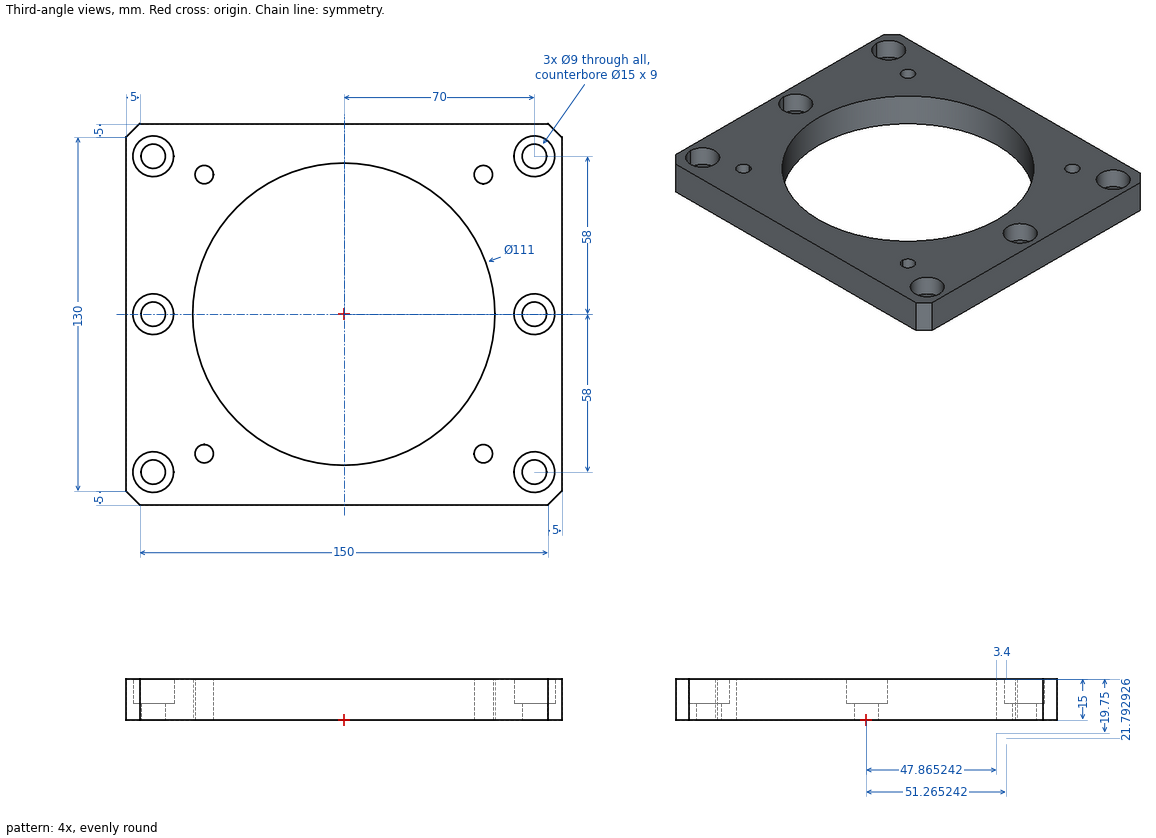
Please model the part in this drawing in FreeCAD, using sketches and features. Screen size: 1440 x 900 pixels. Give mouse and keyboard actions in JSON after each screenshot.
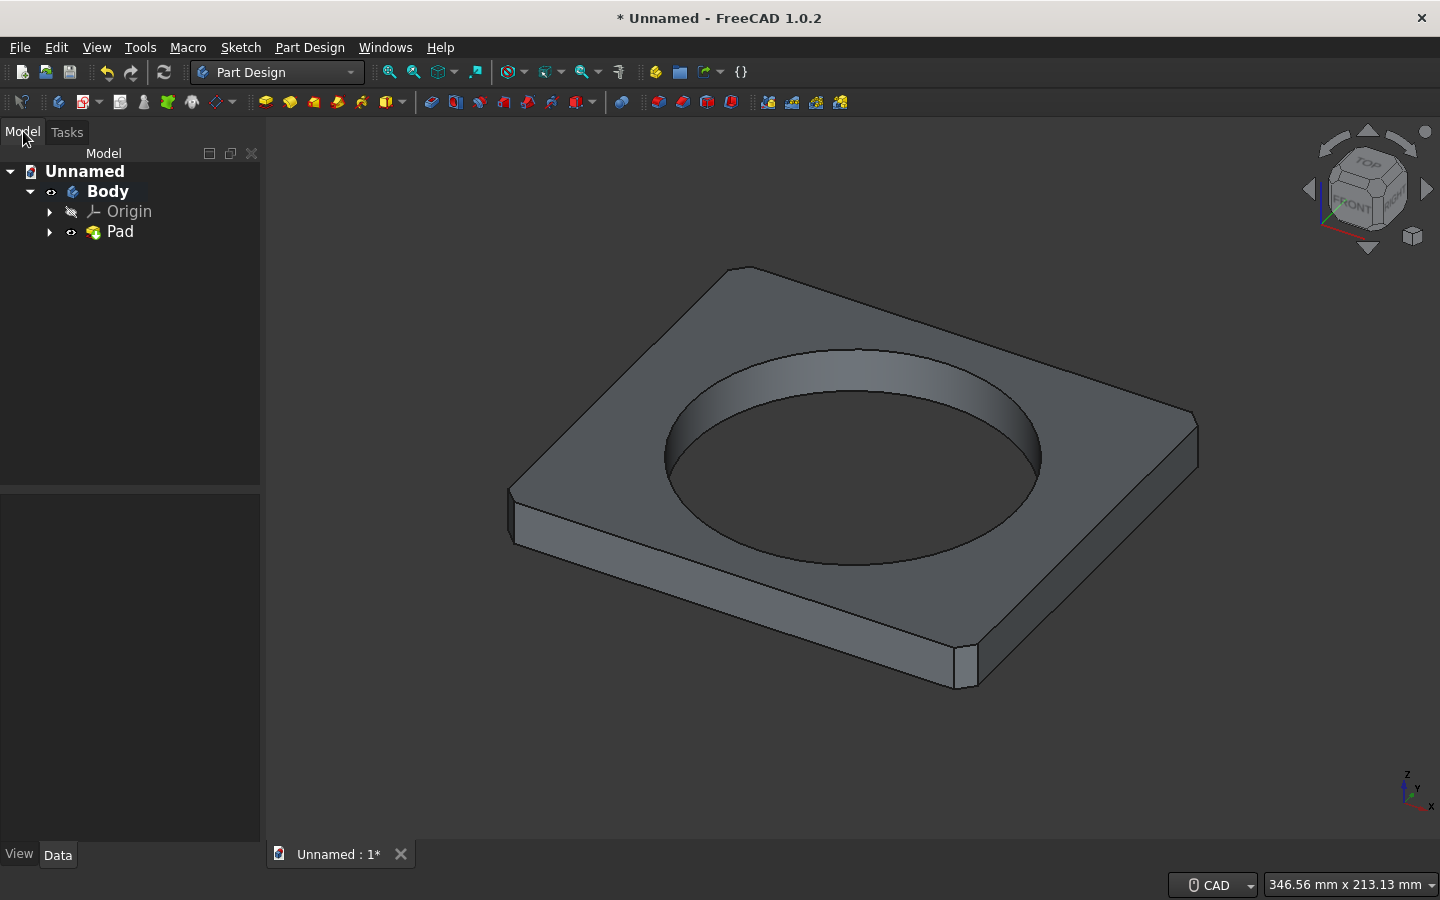
{"action": "left_click", "coordinate": [50, 212]}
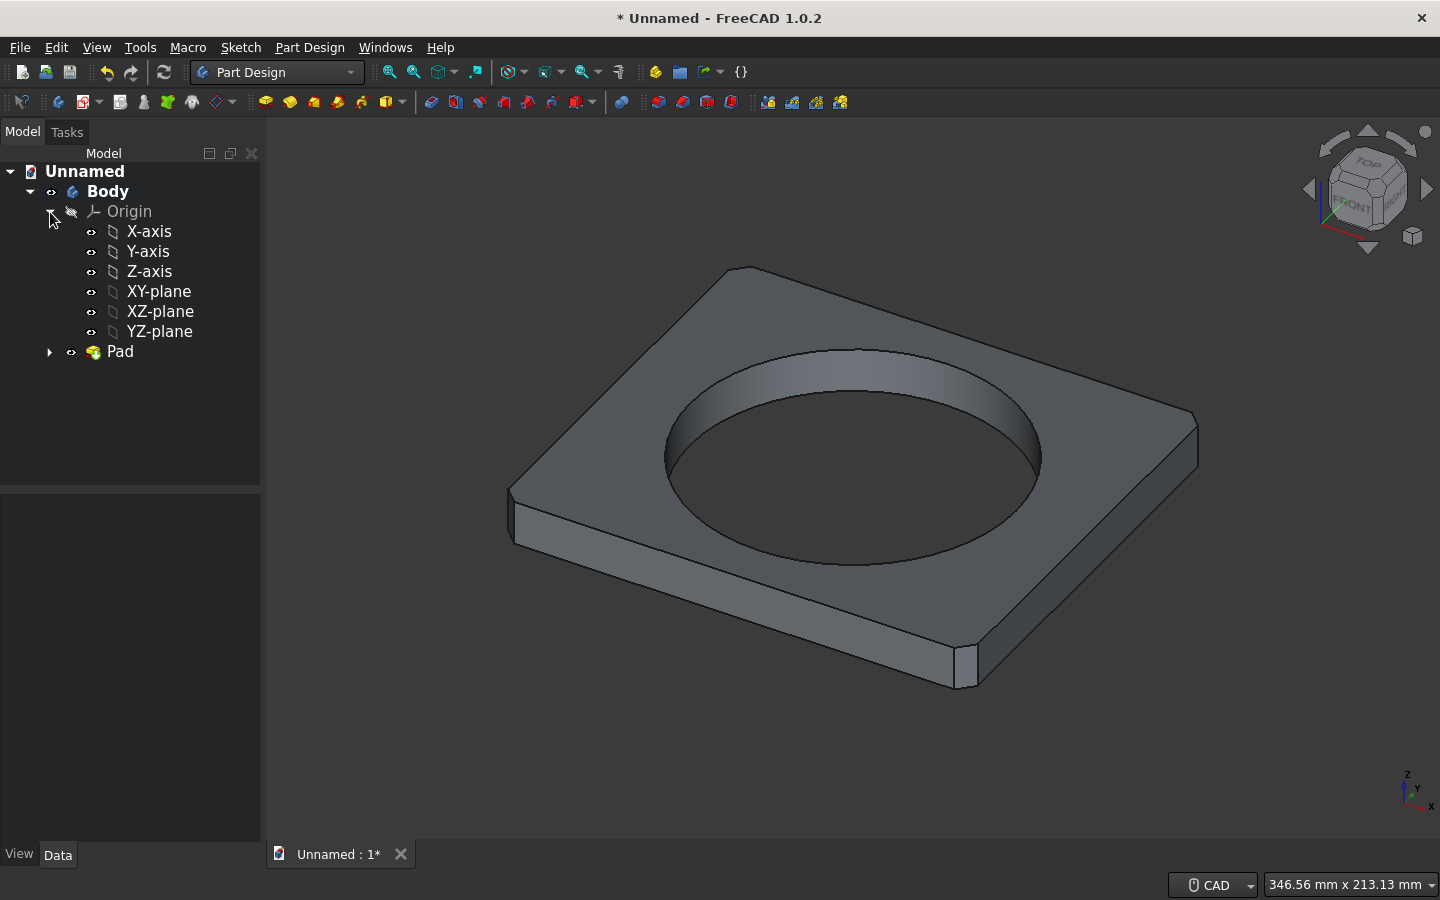
{"action": "left_click", "coordinate": [136, 332]}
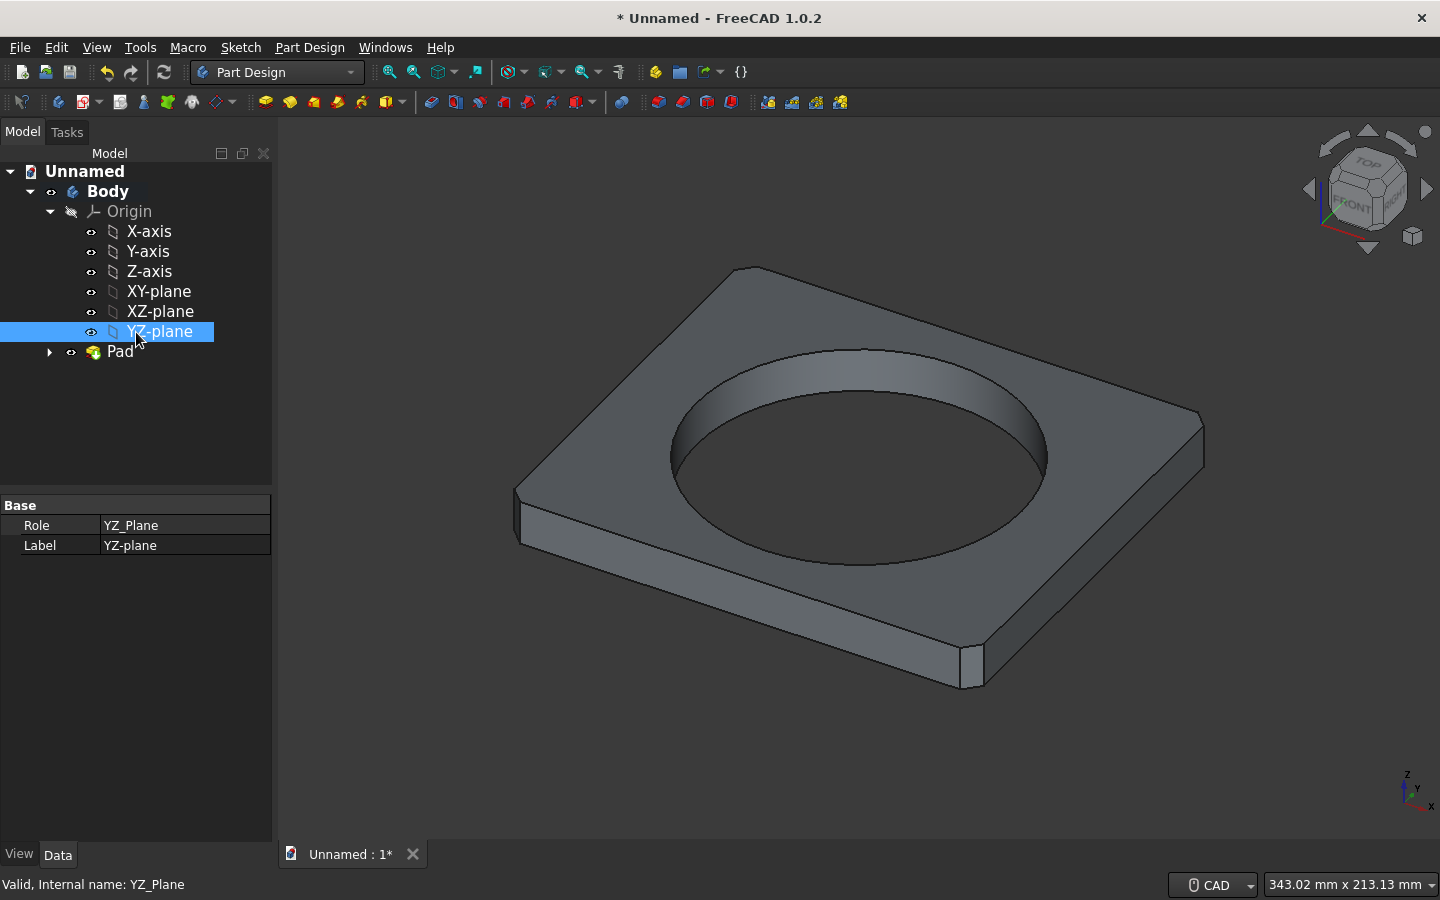
{"action": "left_click", "coordinate": [216, 102]}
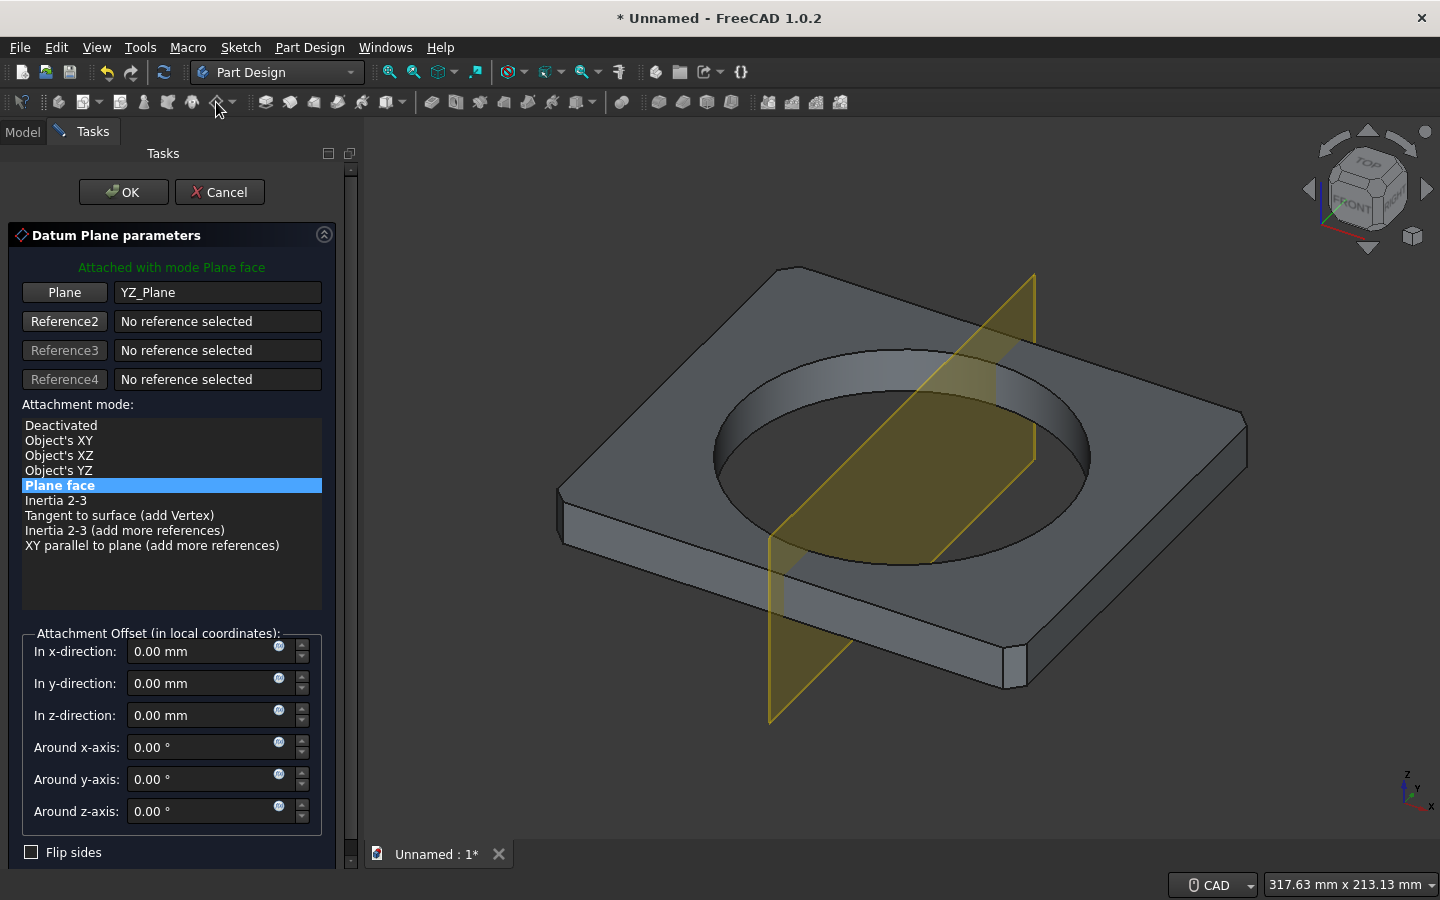
{"action": "triple_click", "coordinate": [210, 715]}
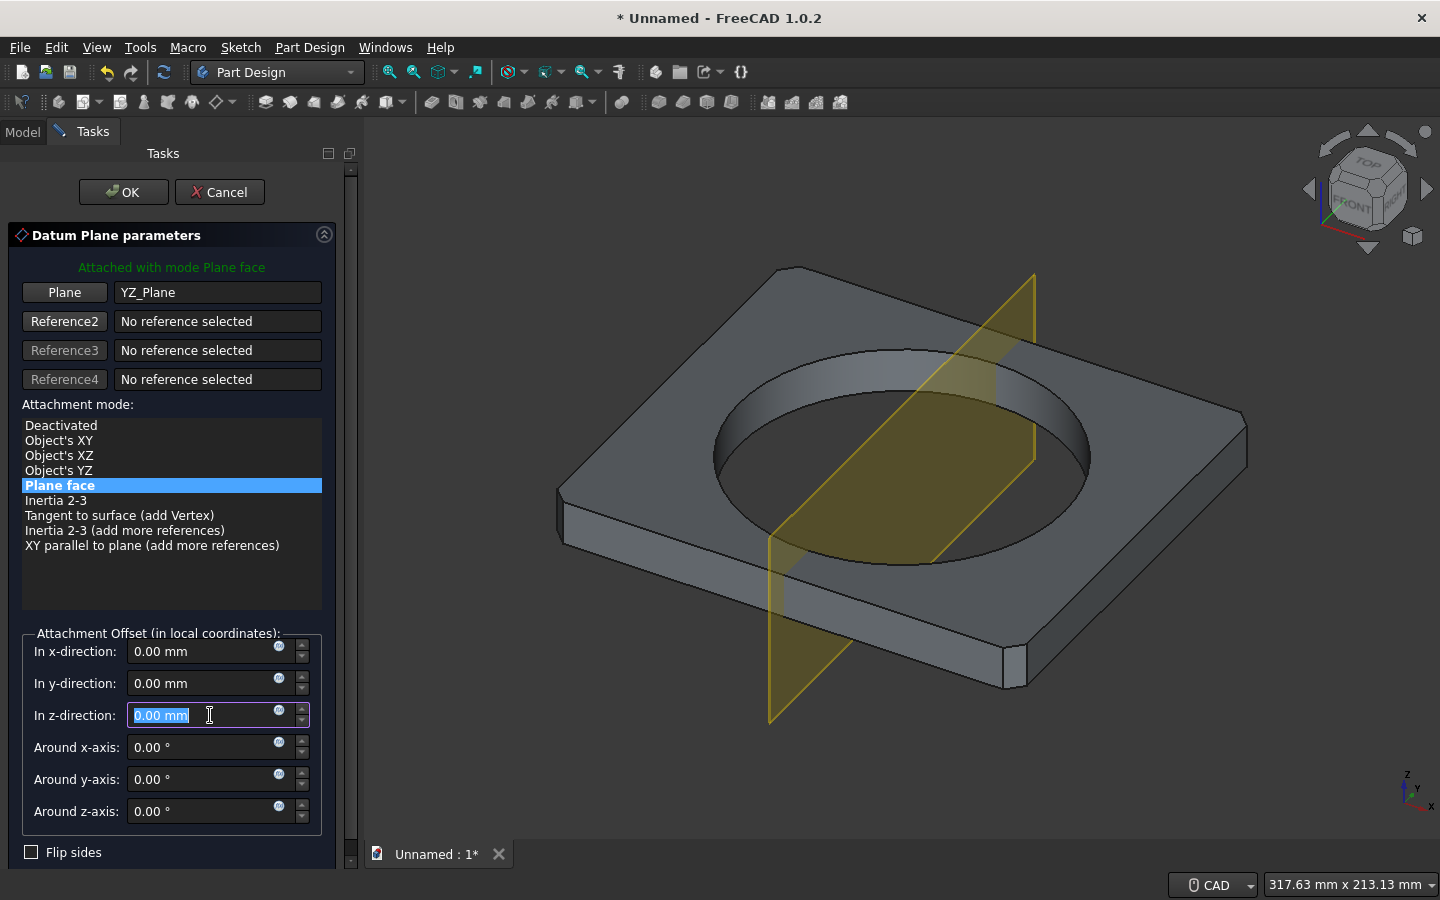
{"action": "type", "text": "51.265242"}
{"action": "key", "text": "Tab"}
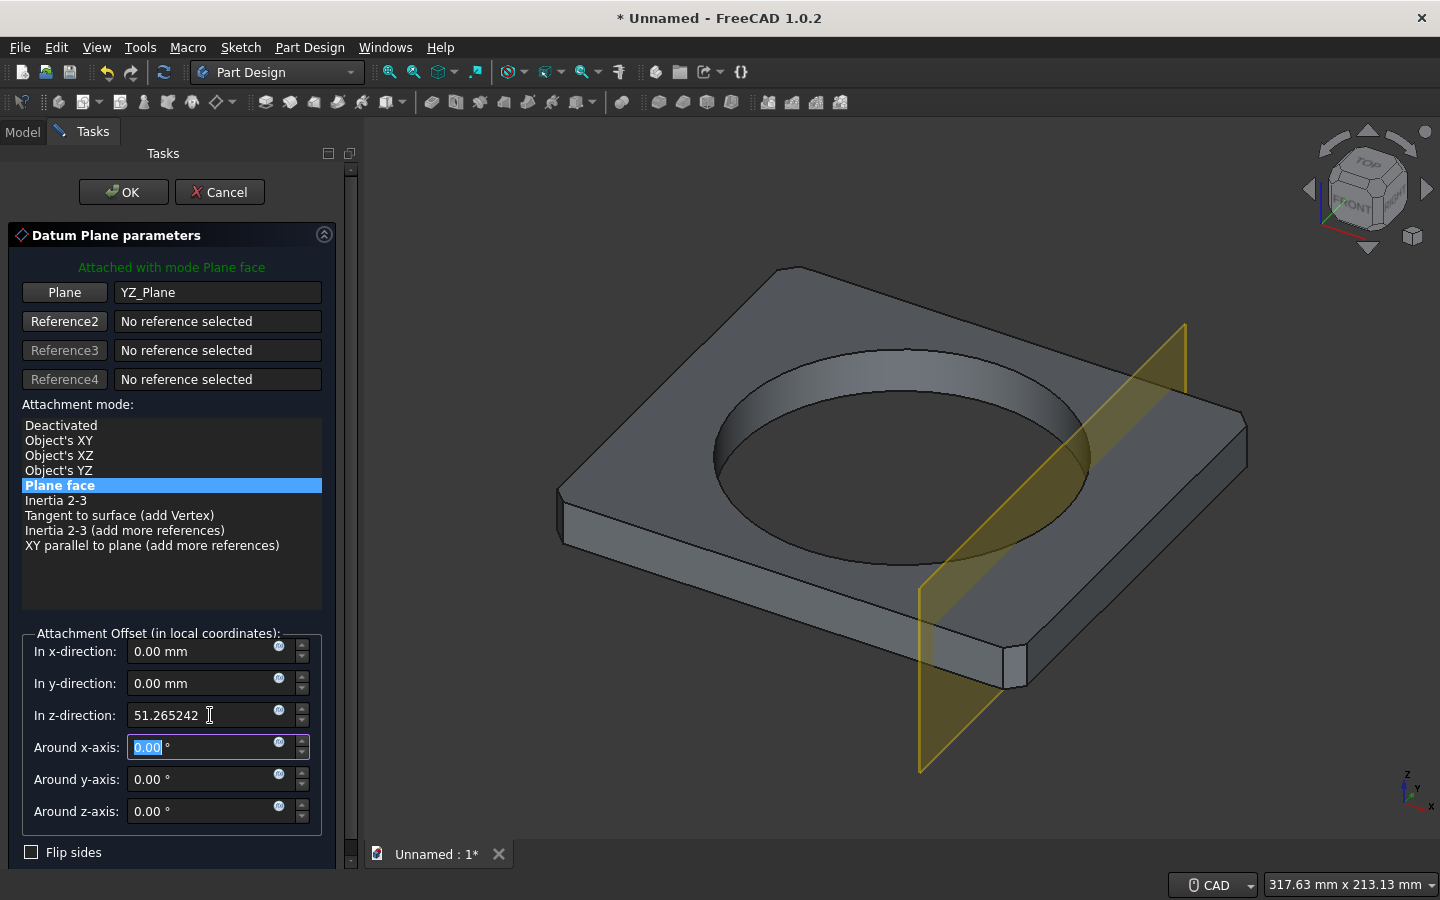
{"action": "left_click", "coordinate": [124, 192]}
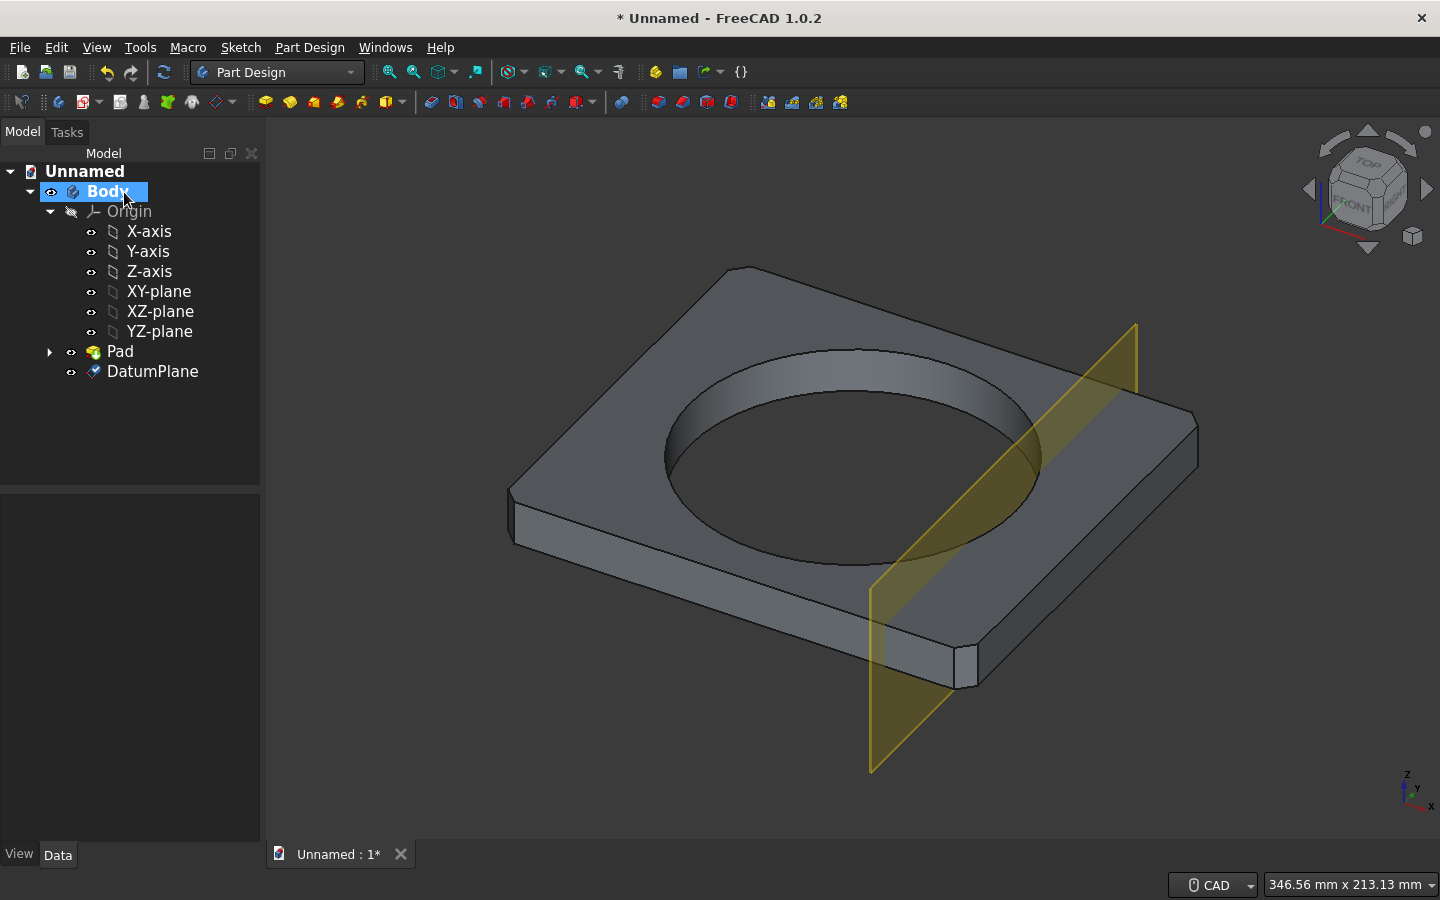
{"action": "left_click", "coordinate": [116, 372]}